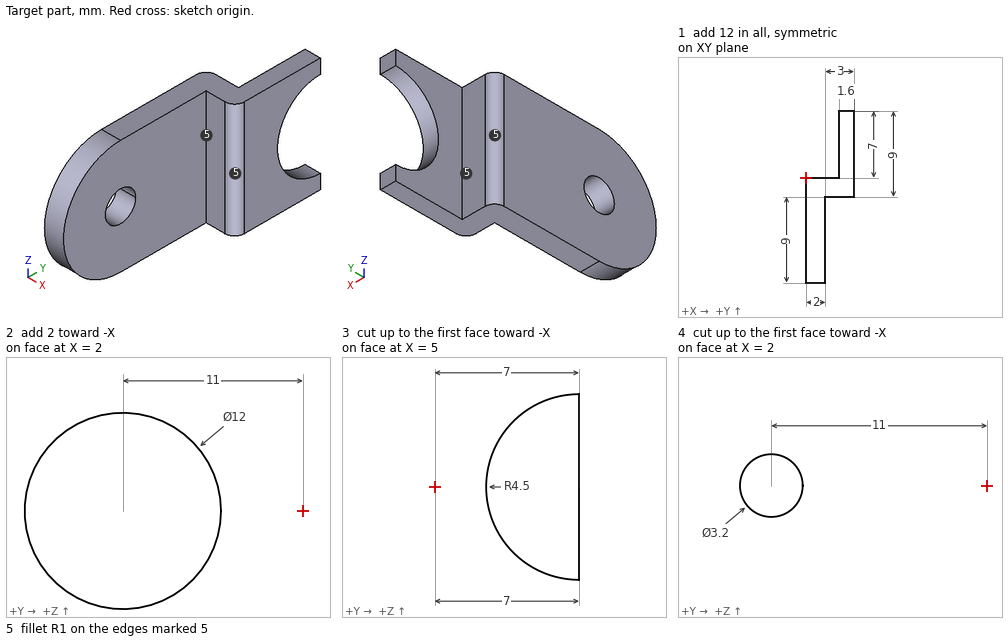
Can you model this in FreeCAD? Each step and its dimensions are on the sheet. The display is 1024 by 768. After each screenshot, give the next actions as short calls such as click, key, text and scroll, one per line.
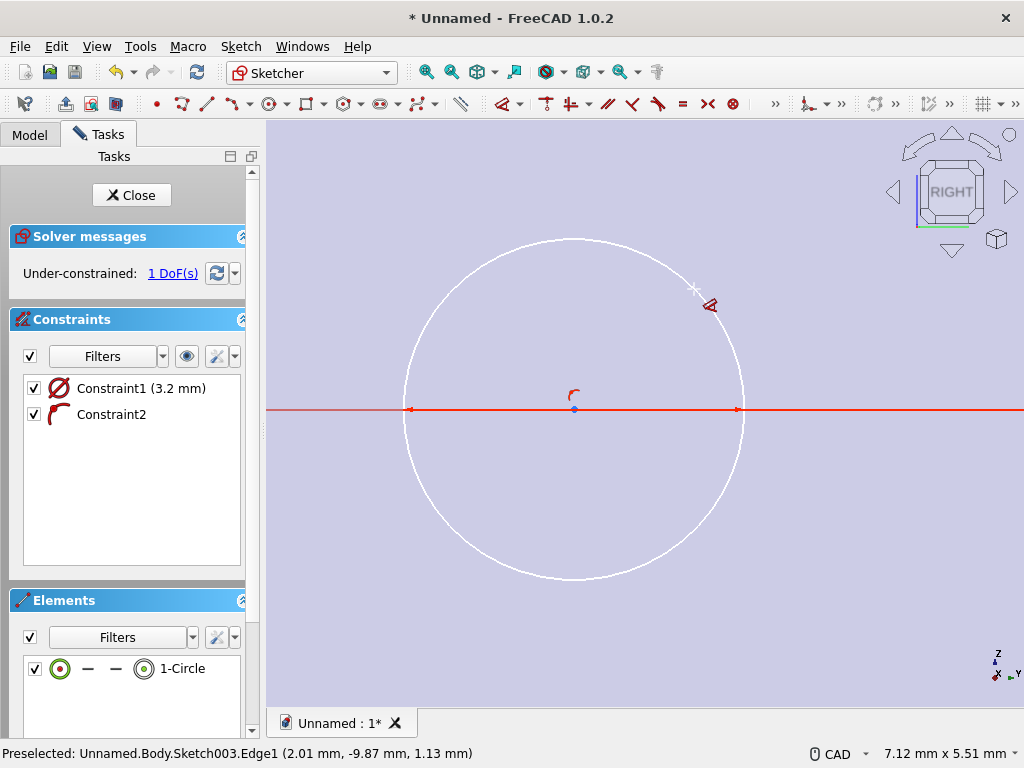
click(574, 410)
click(717, 444)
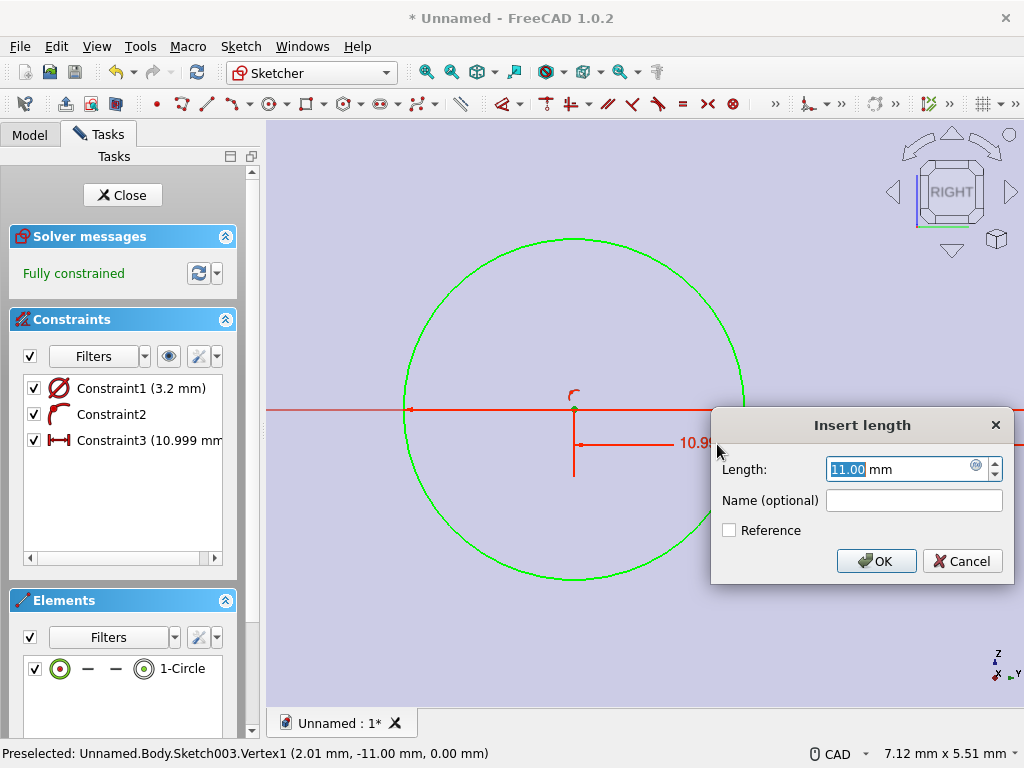
text(11)
key(Return)
key(Escape)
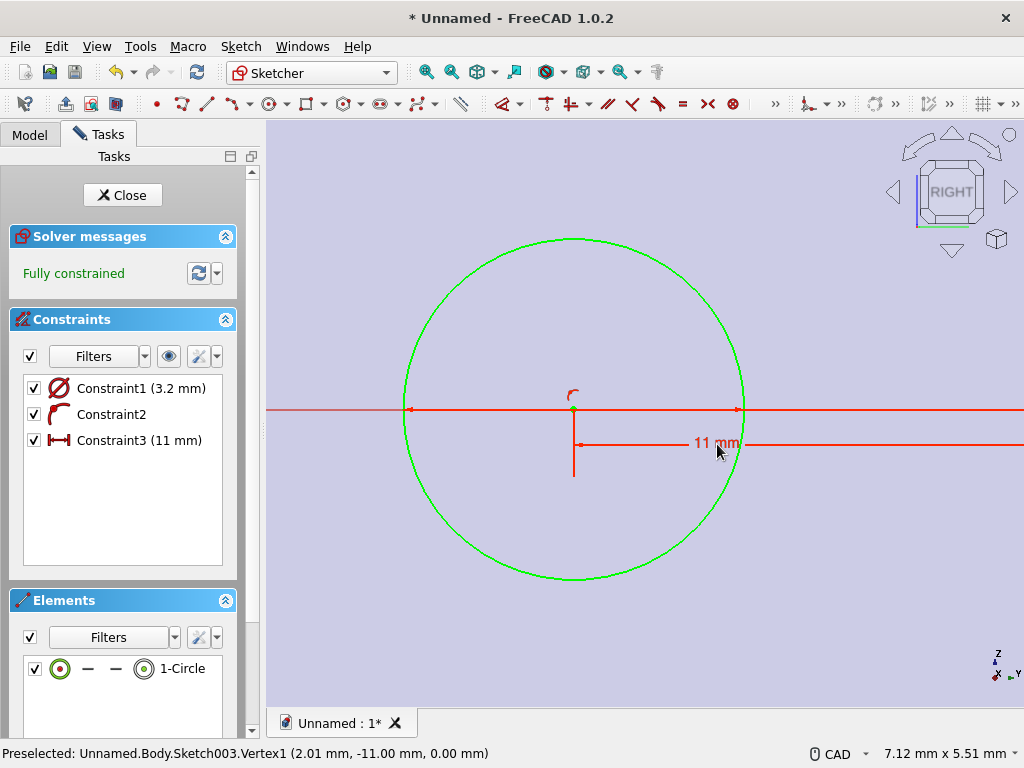
click(123, 195)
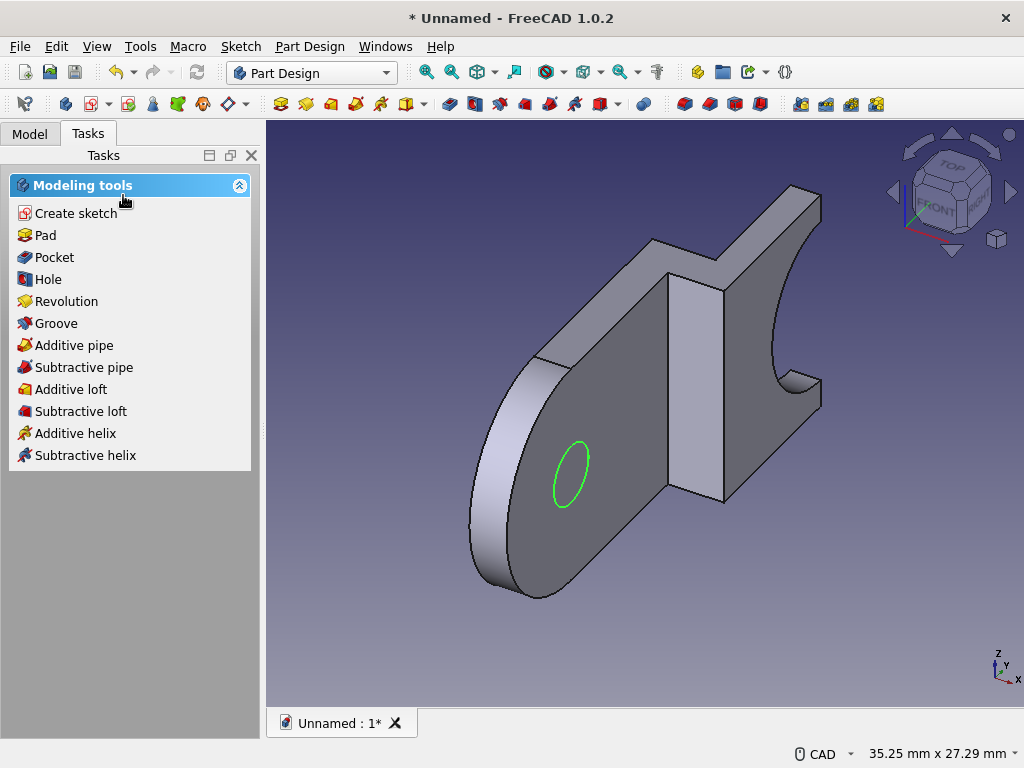
click(450, 104)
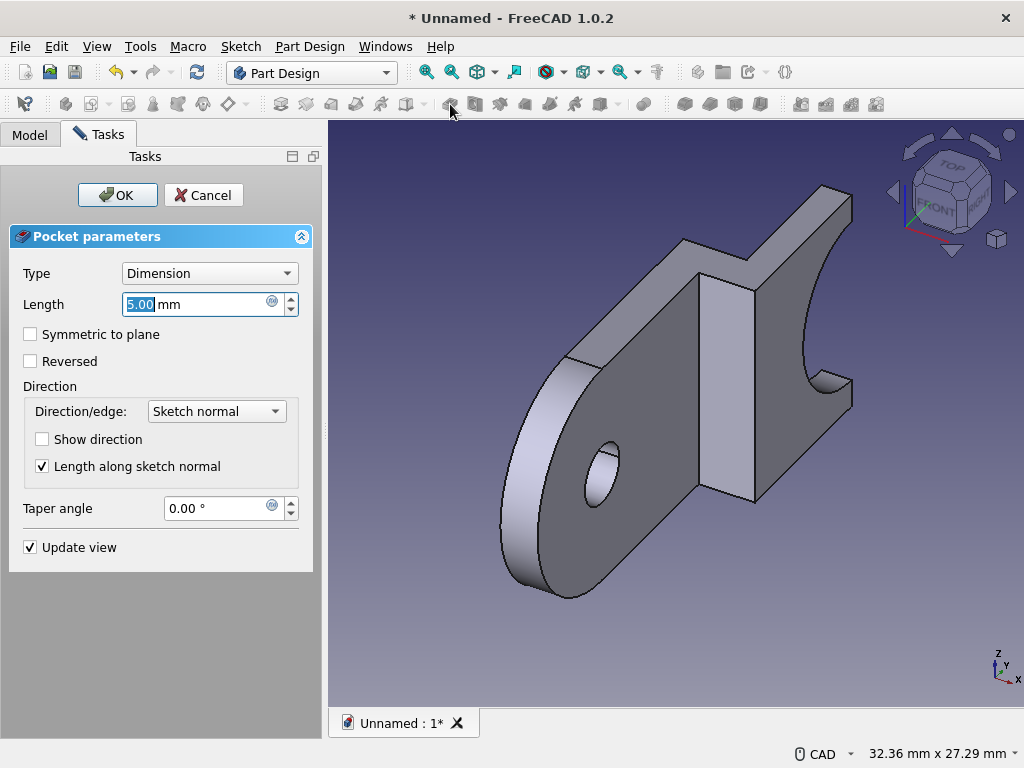
click(210, 274)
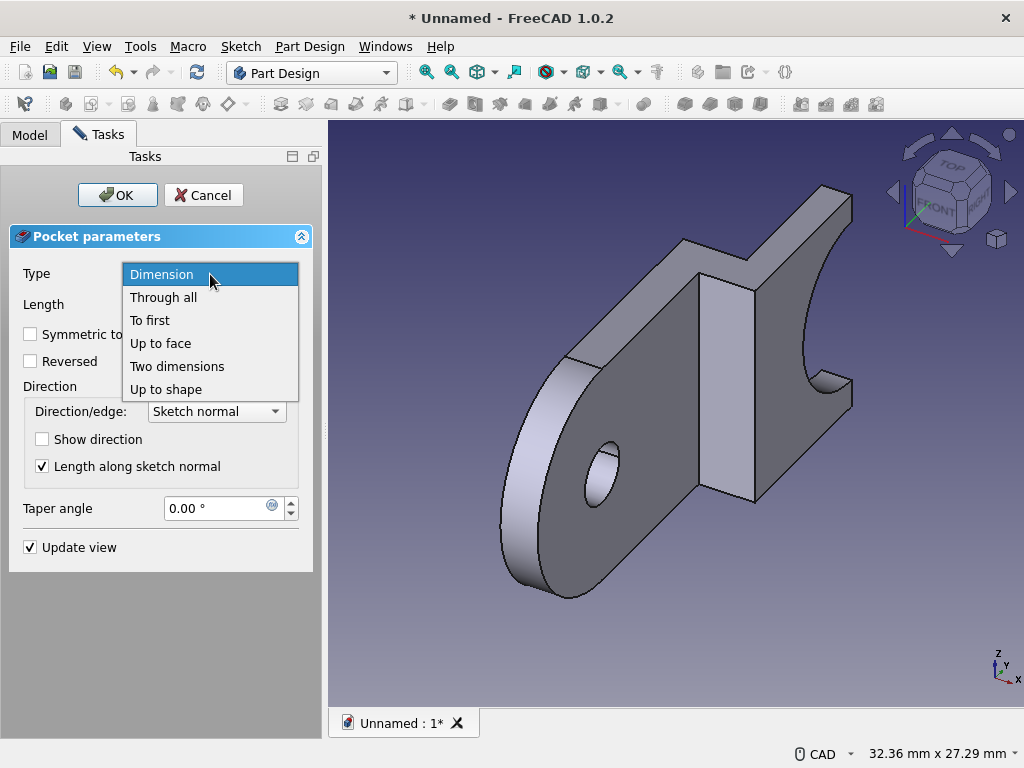
click(208, 320)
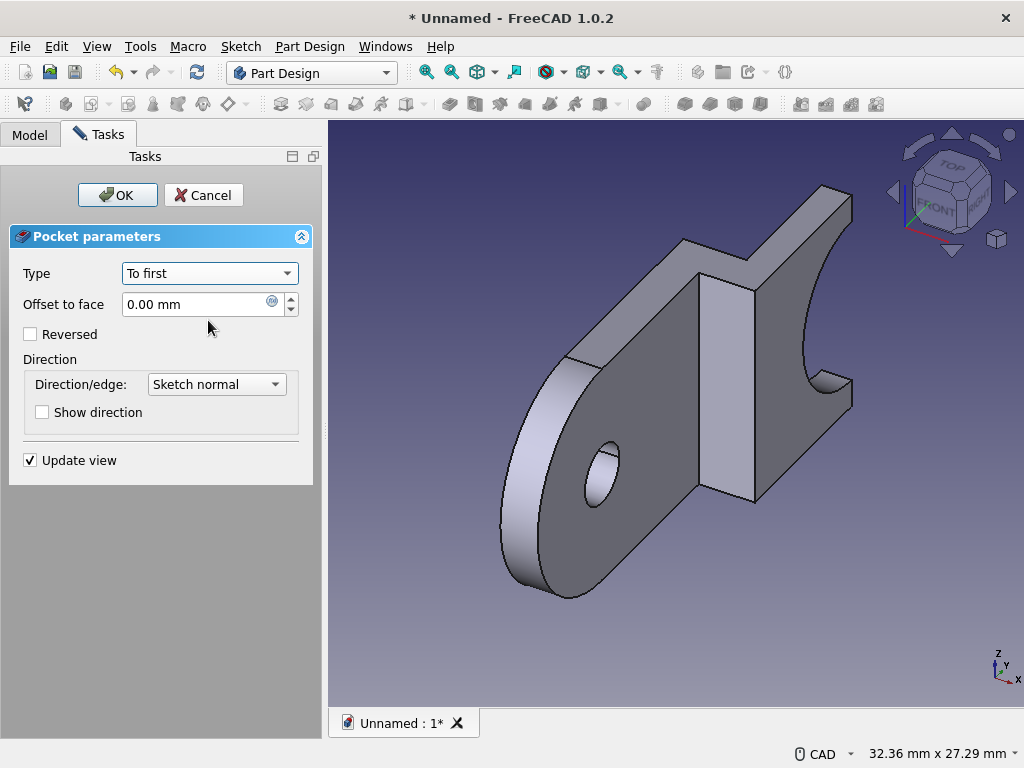
click(118, 195)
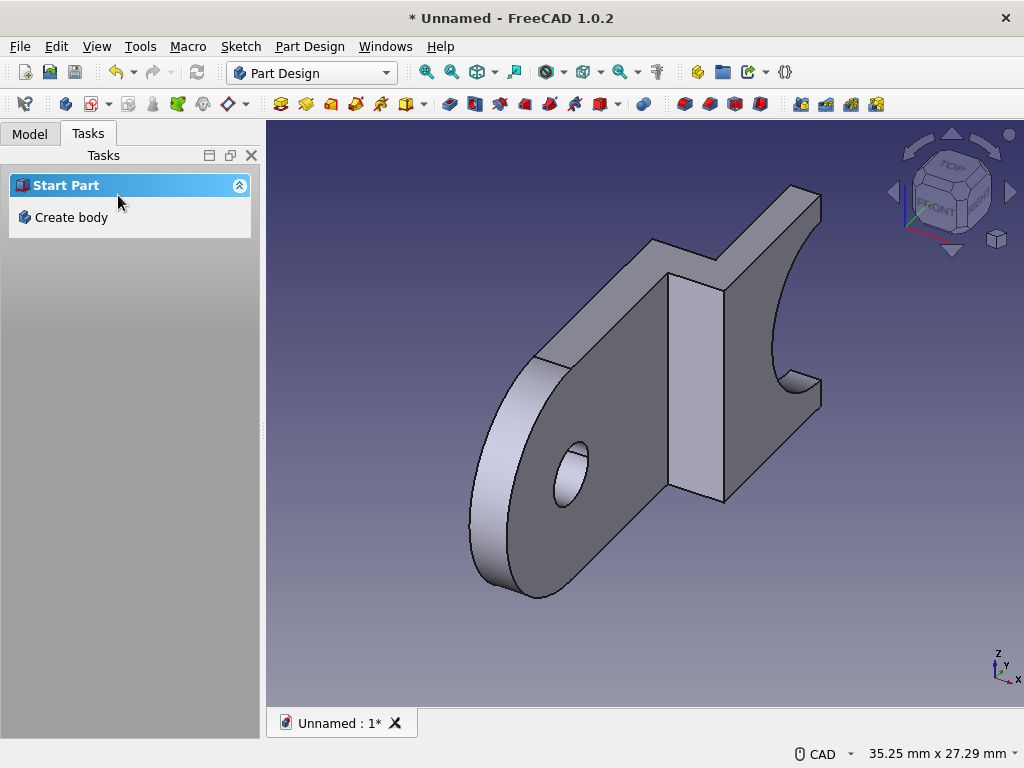
click(724, 396)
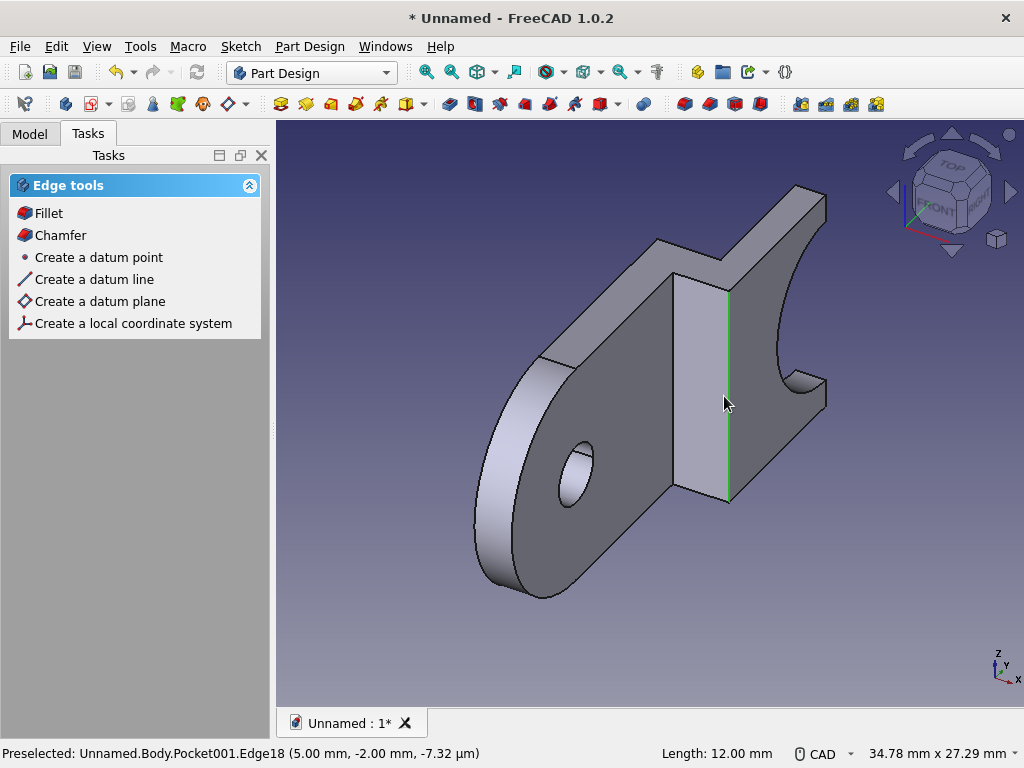
key(0)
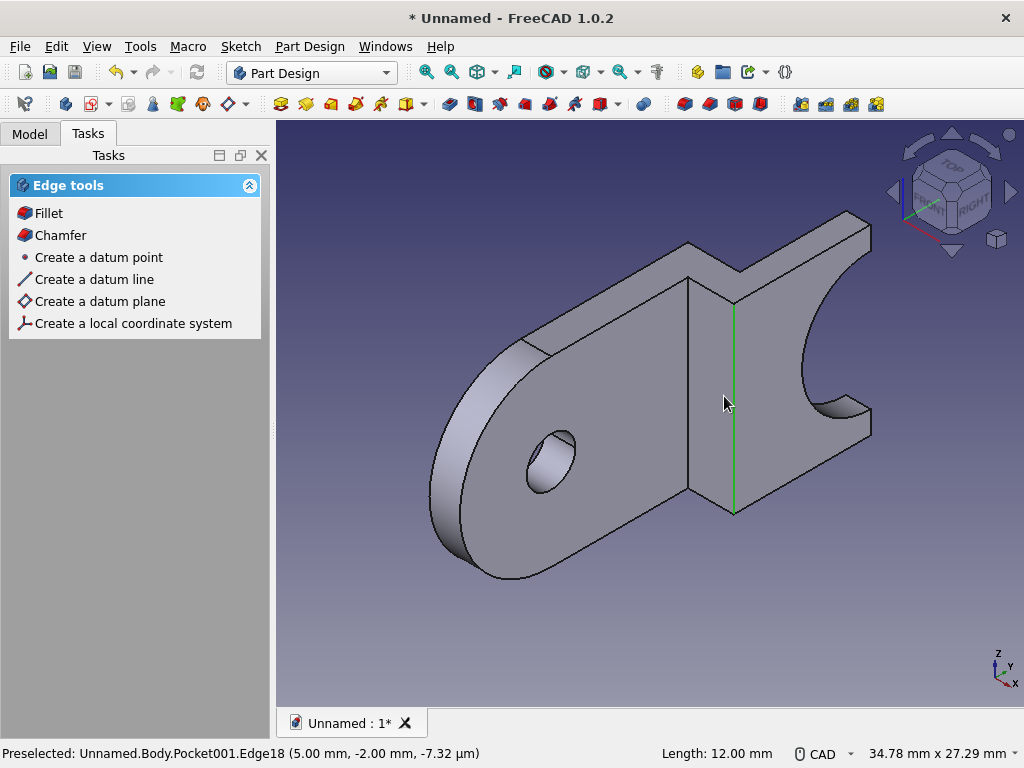
key(2)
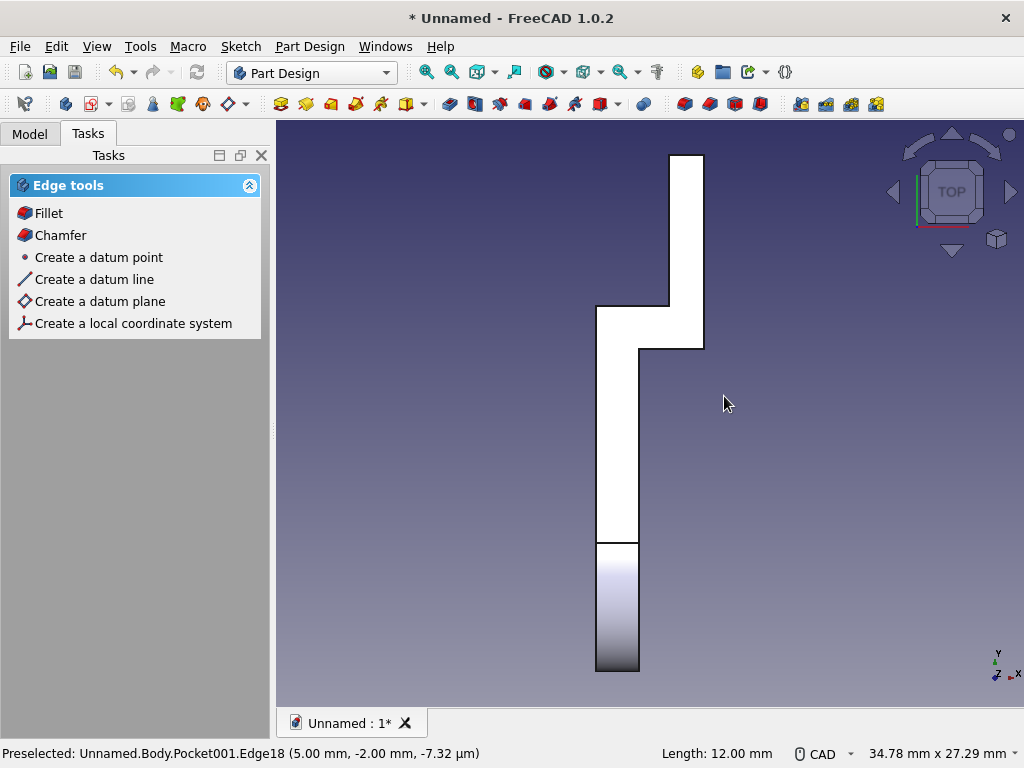
key(1)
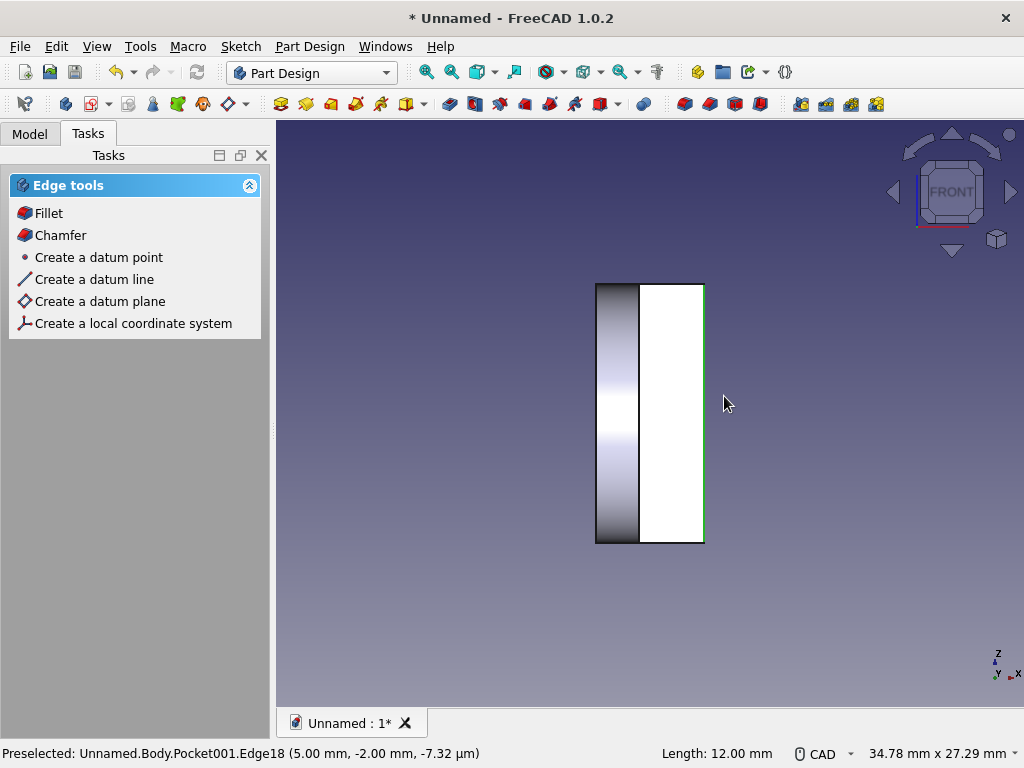
key(v)
key(f)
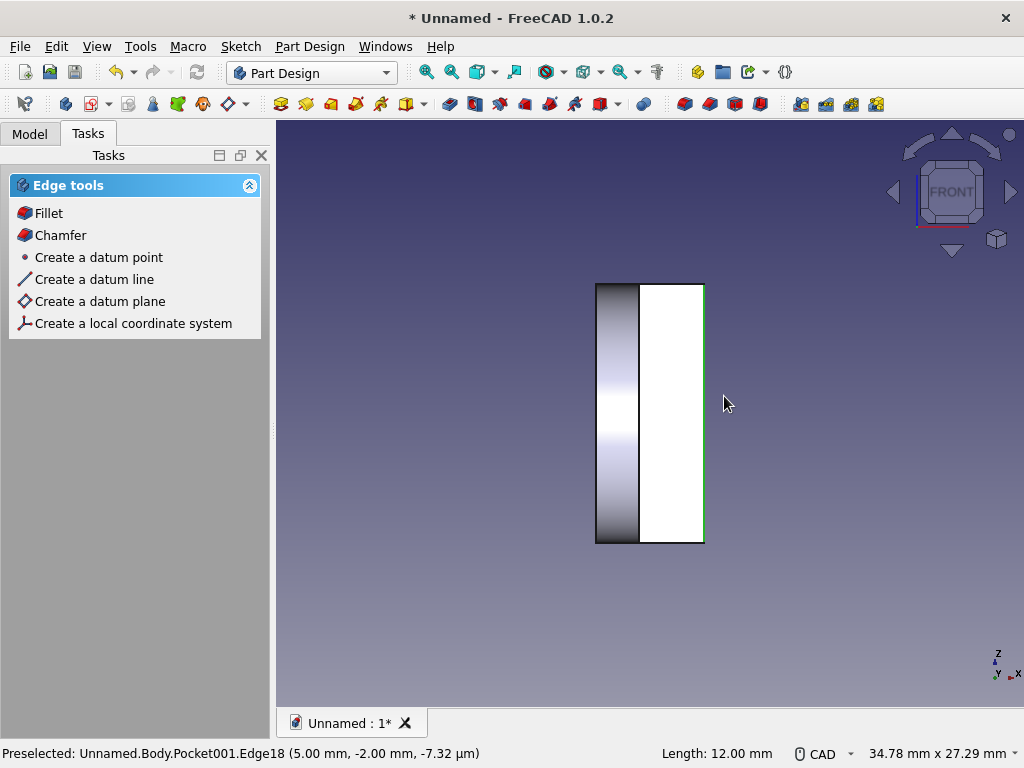
key(3)